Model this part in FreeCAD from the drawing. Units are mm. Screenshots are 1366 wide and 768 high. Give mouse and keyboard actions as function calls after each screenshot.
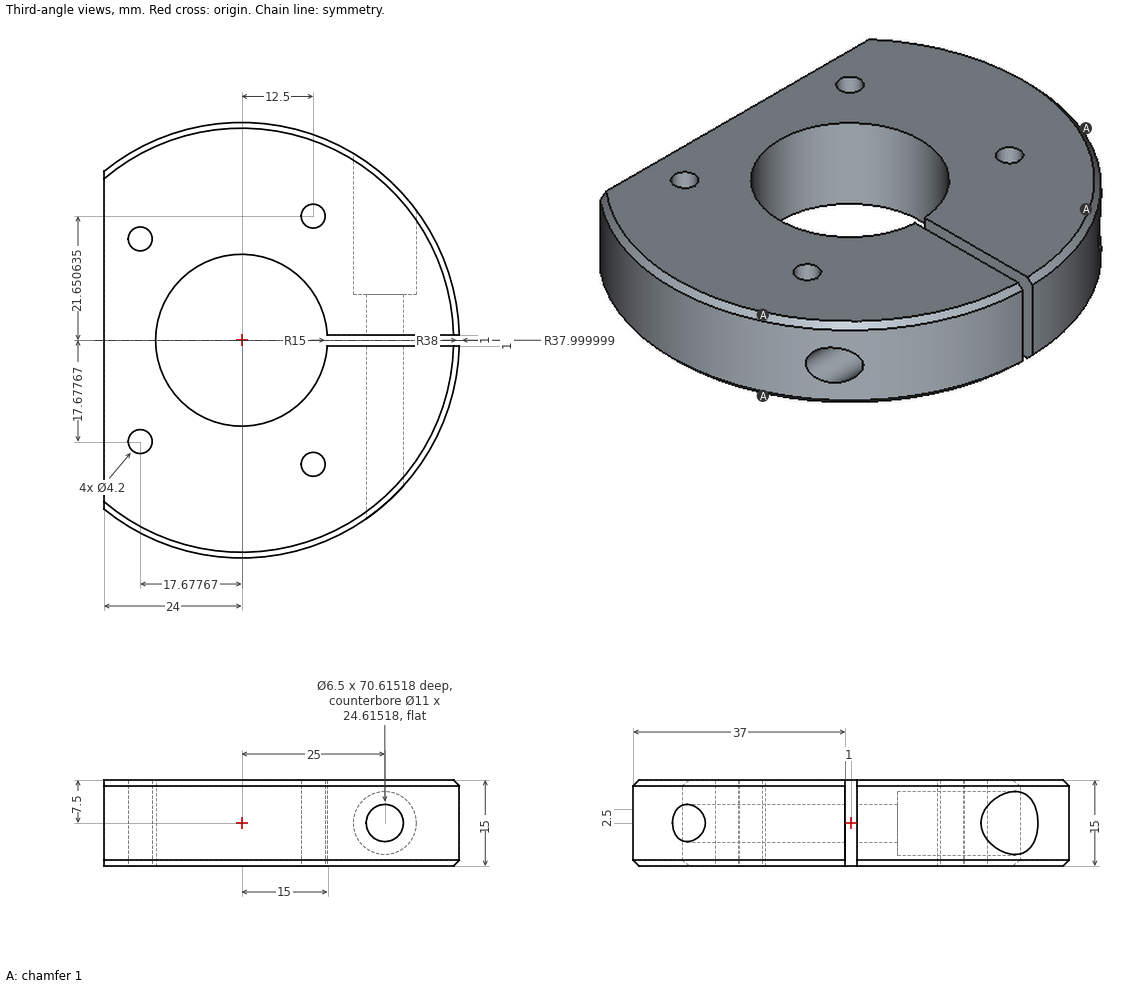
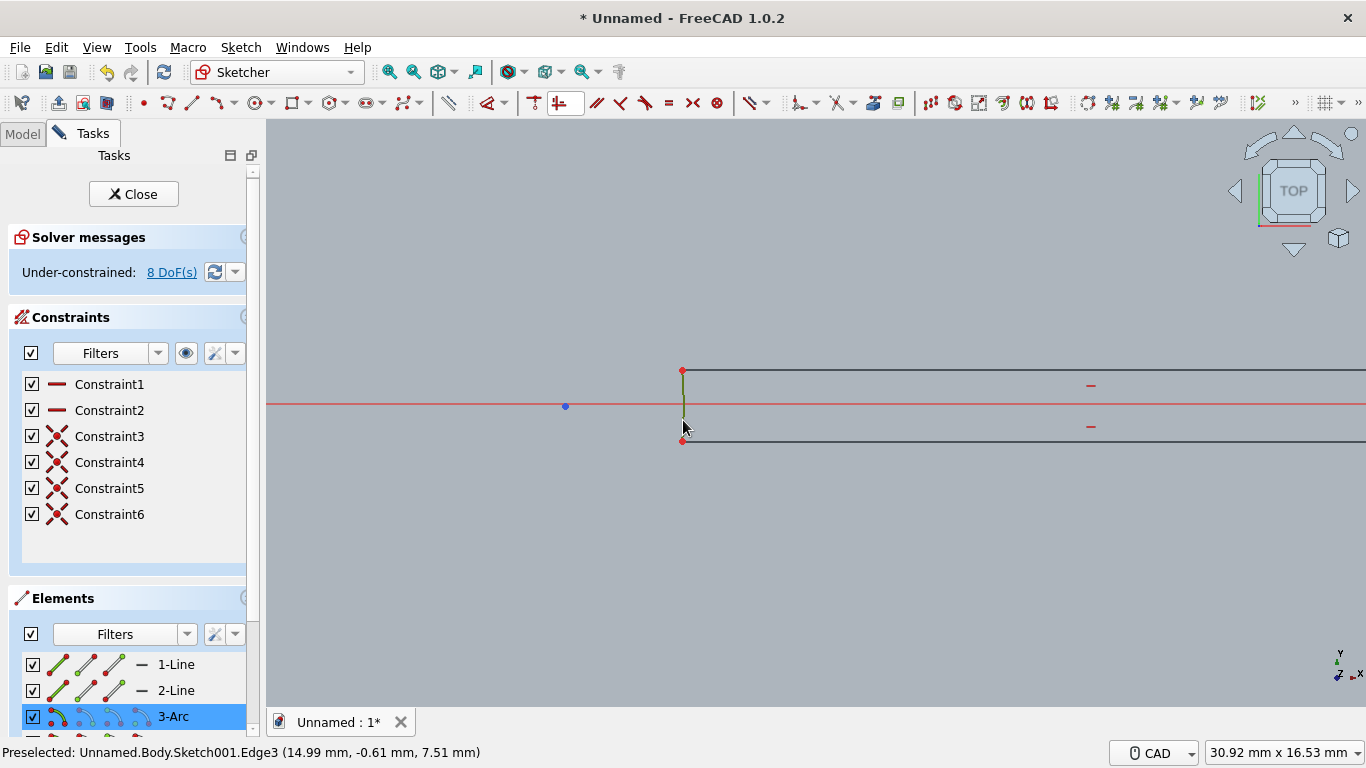
scroll(683, 420, down, 4)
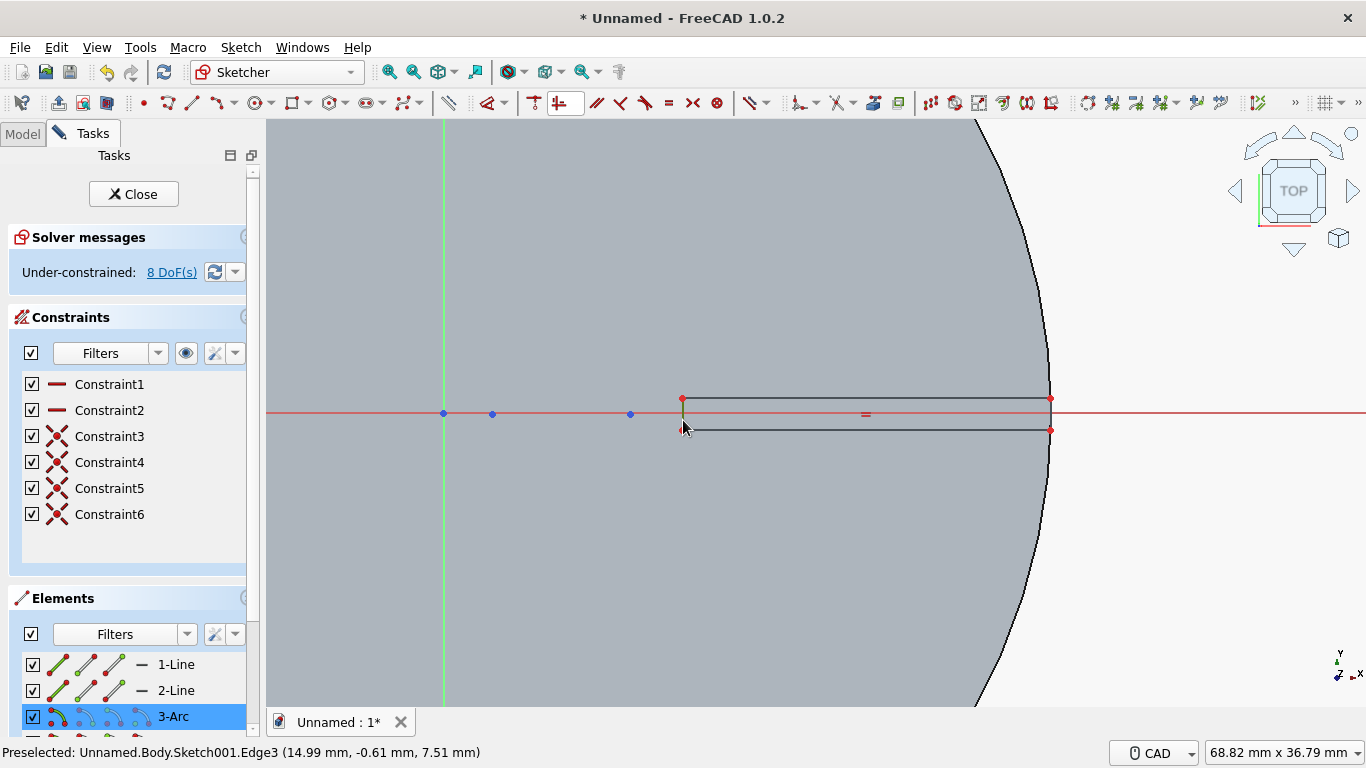
scroll(1051, 420, up, 4)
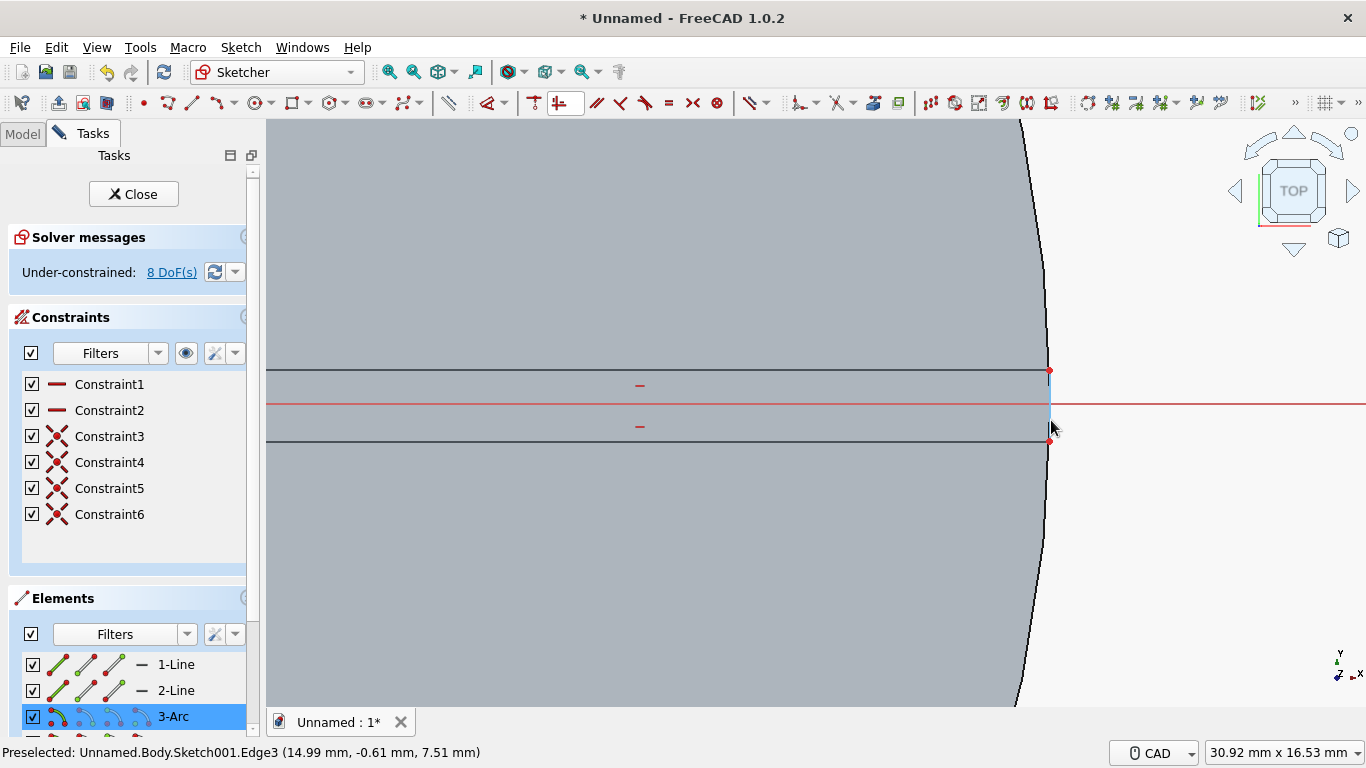
click(1050, 420)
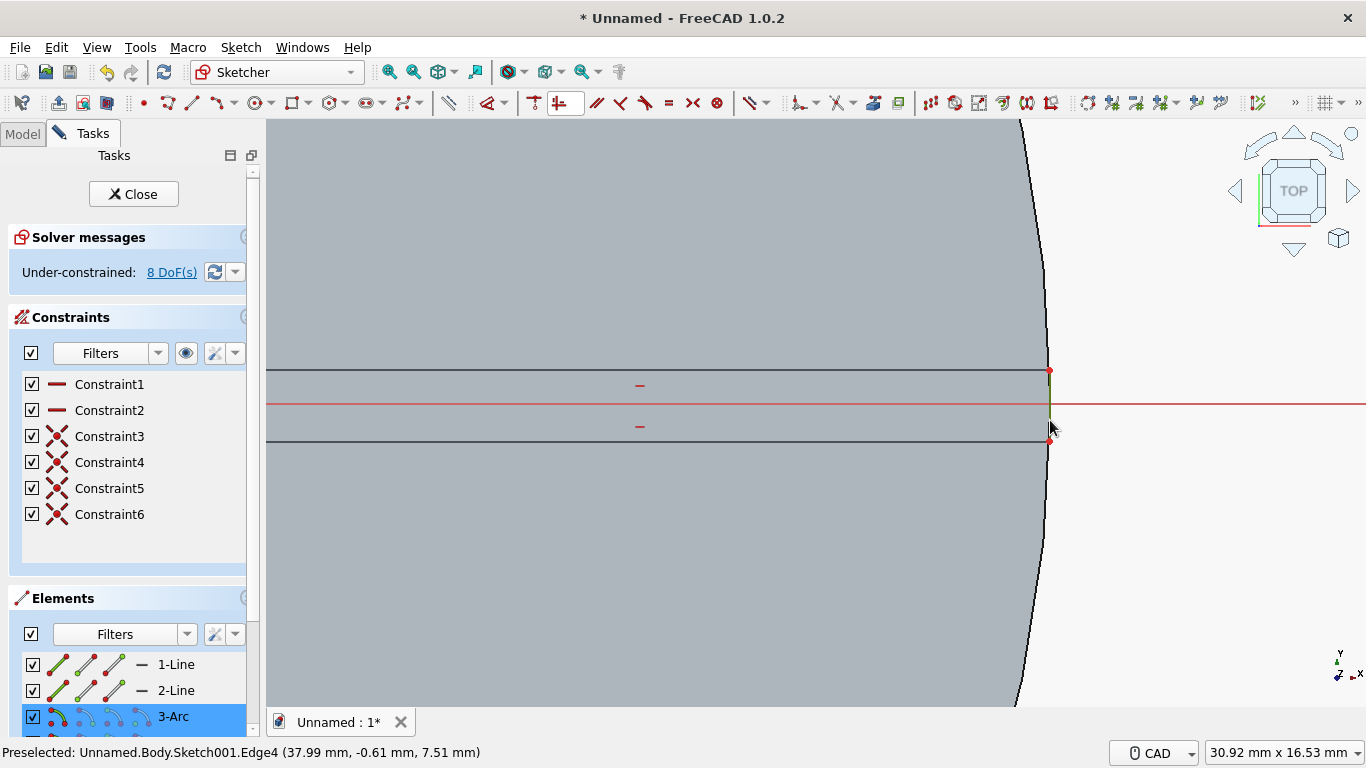
click(534, 104)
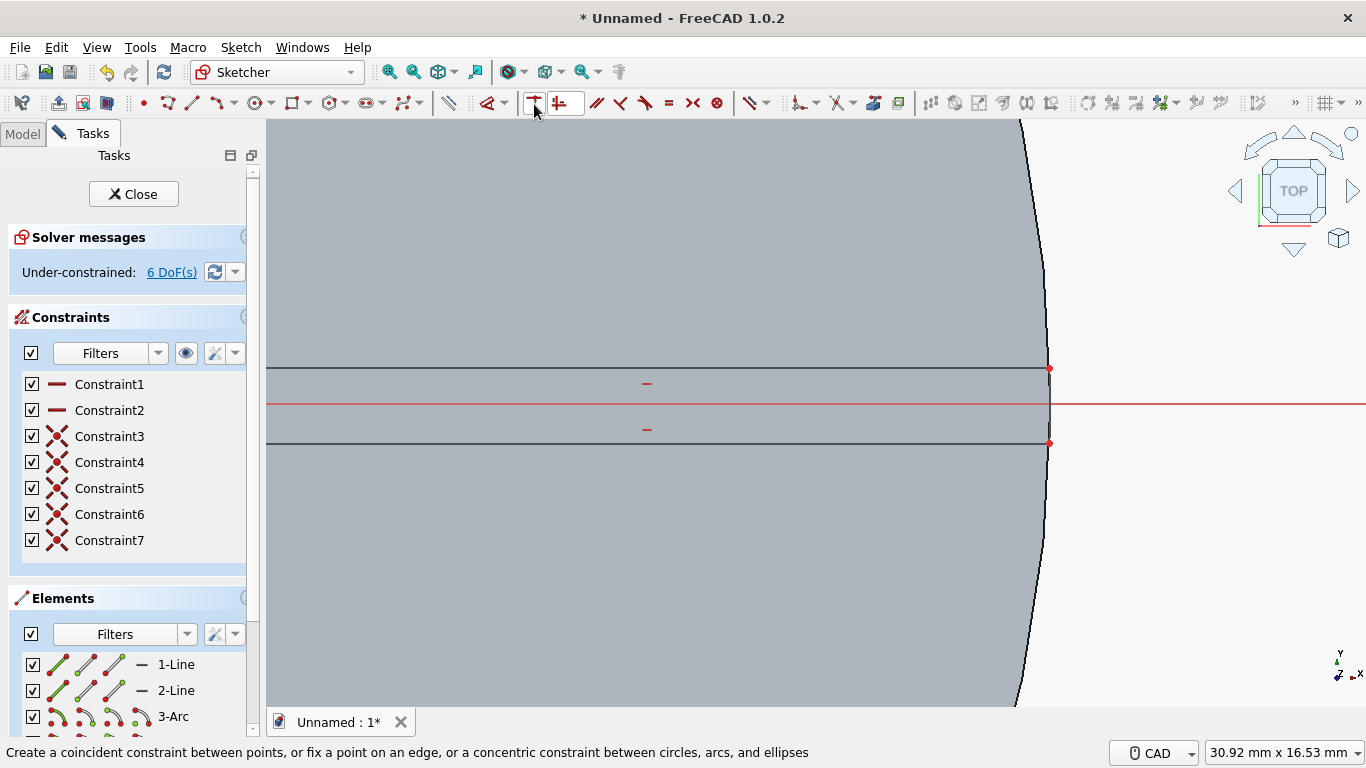
scroll(1052, 420, down, 4)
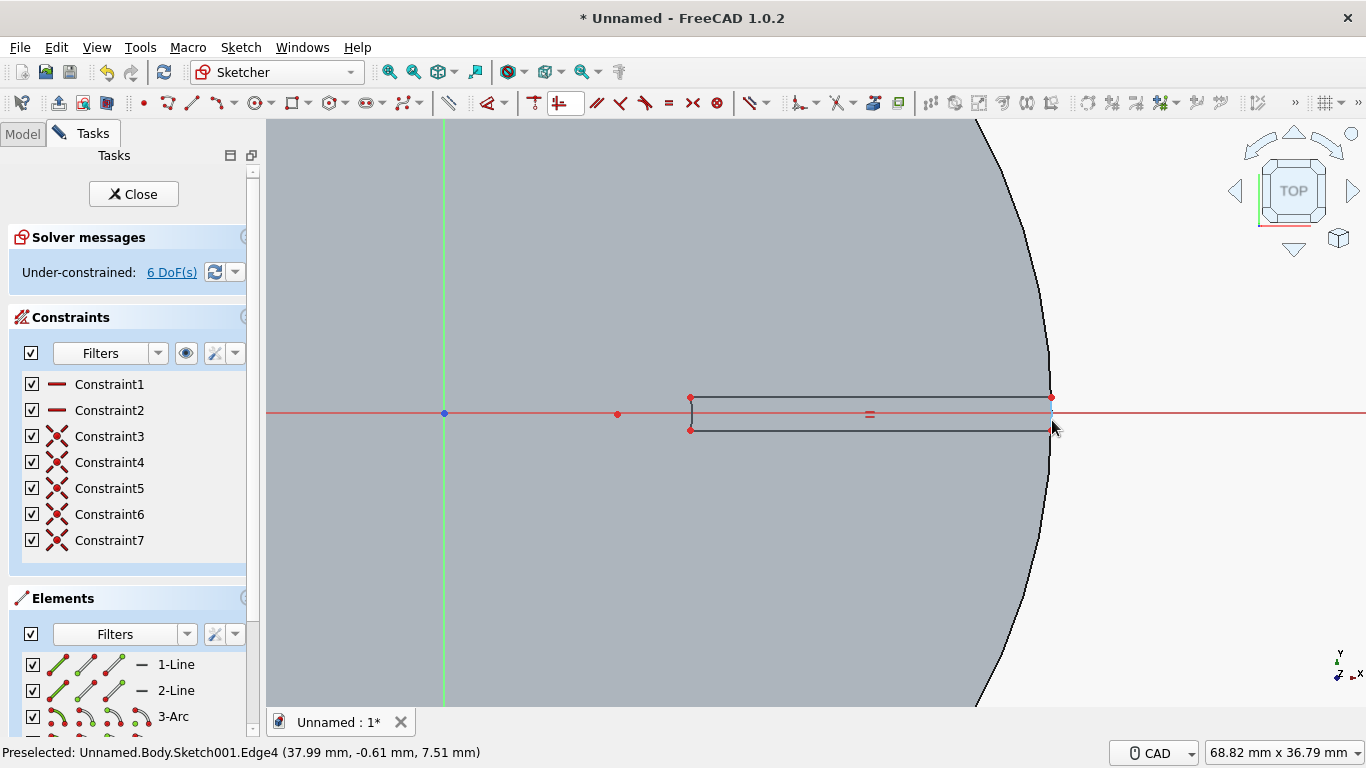
drag(434, 403, 628, 424)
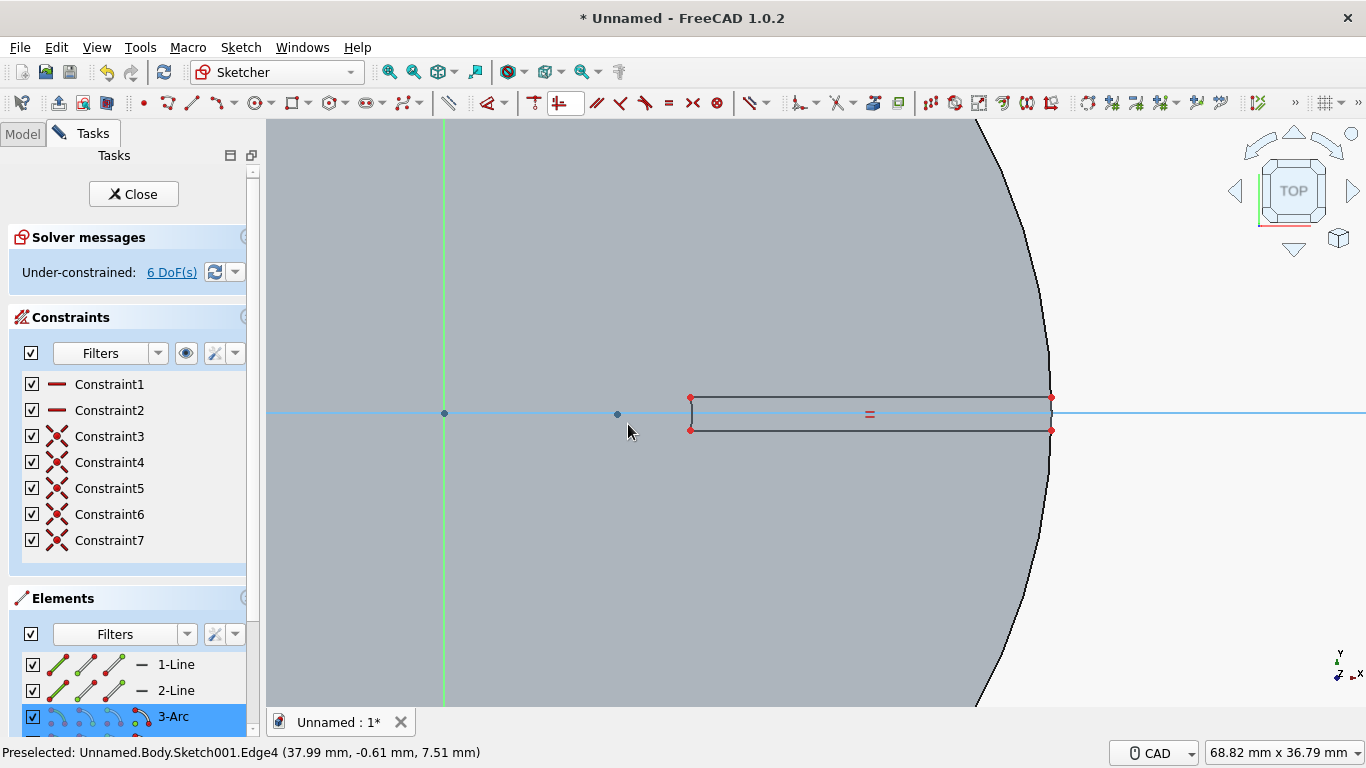
click(534, 104)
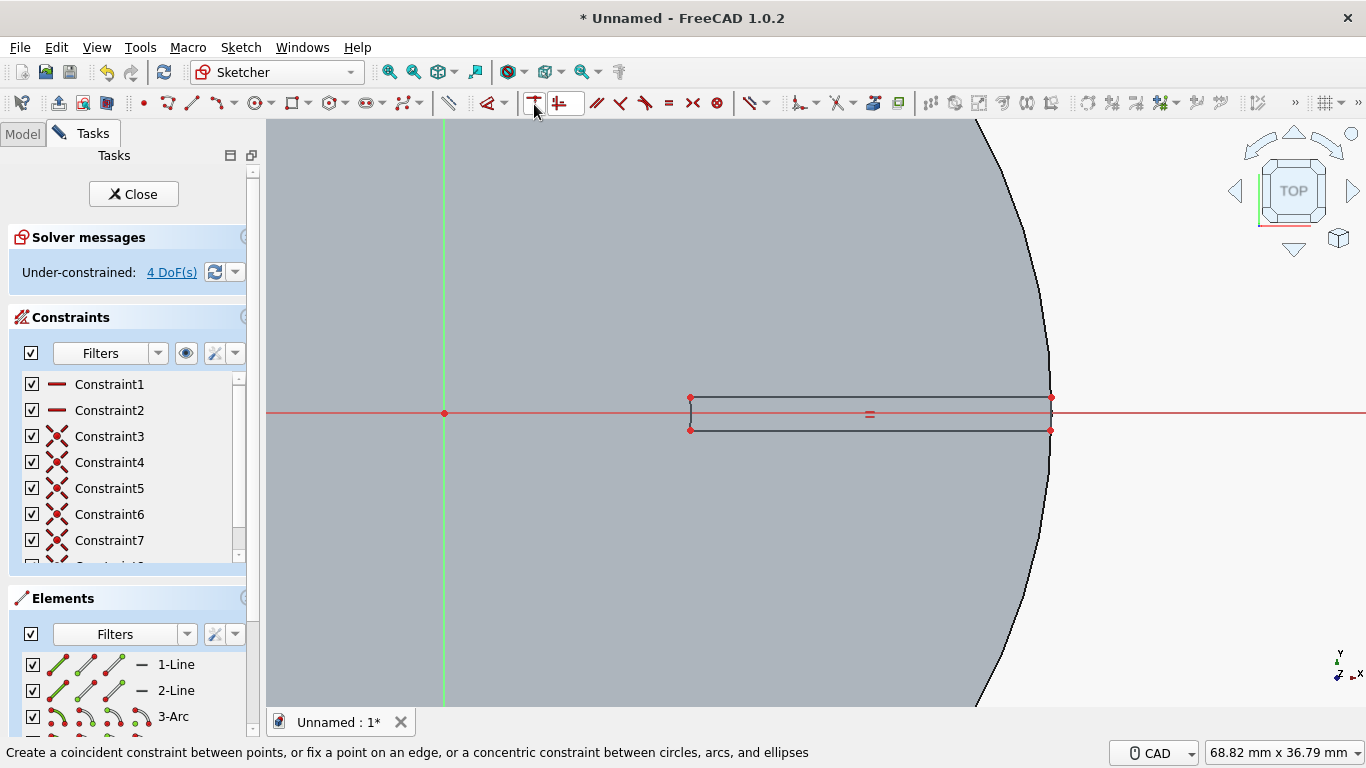
click(488, 104)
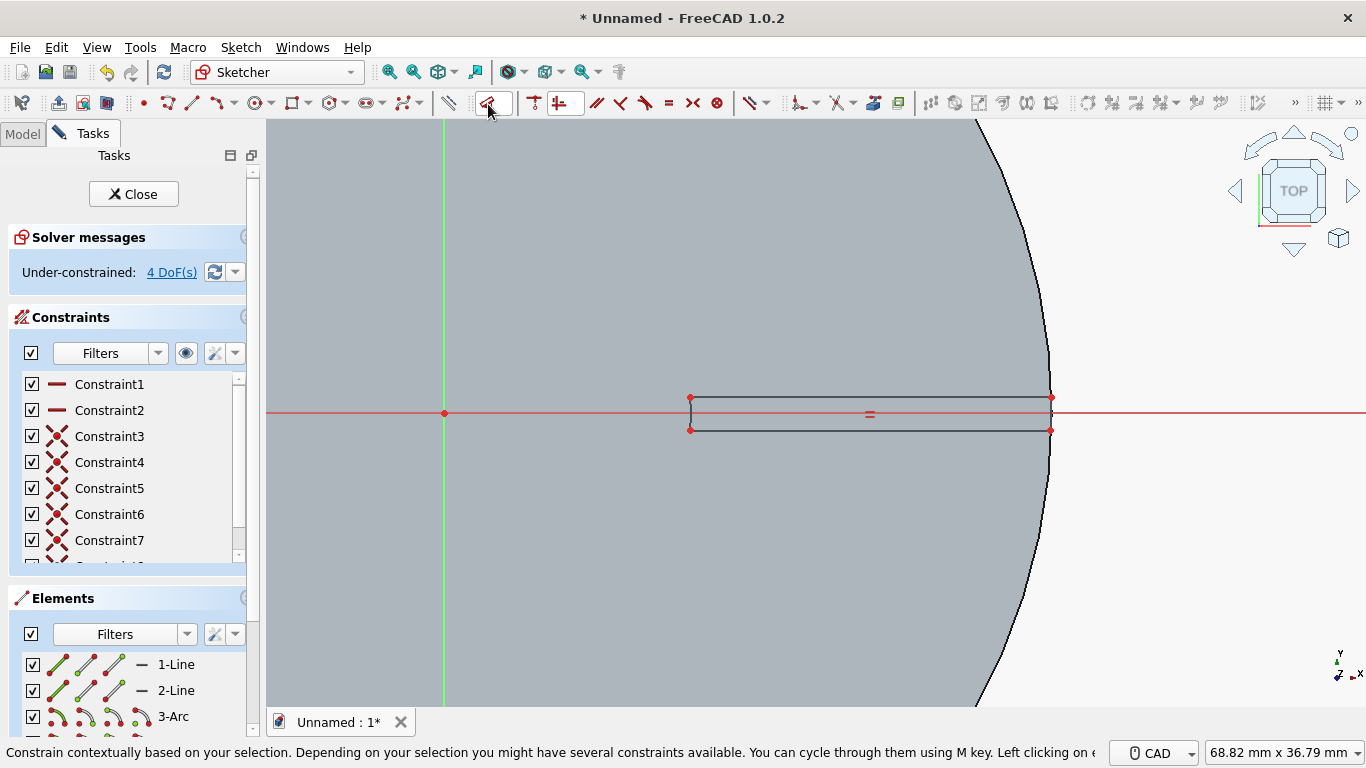
click(691, 414)
click(688, 548)